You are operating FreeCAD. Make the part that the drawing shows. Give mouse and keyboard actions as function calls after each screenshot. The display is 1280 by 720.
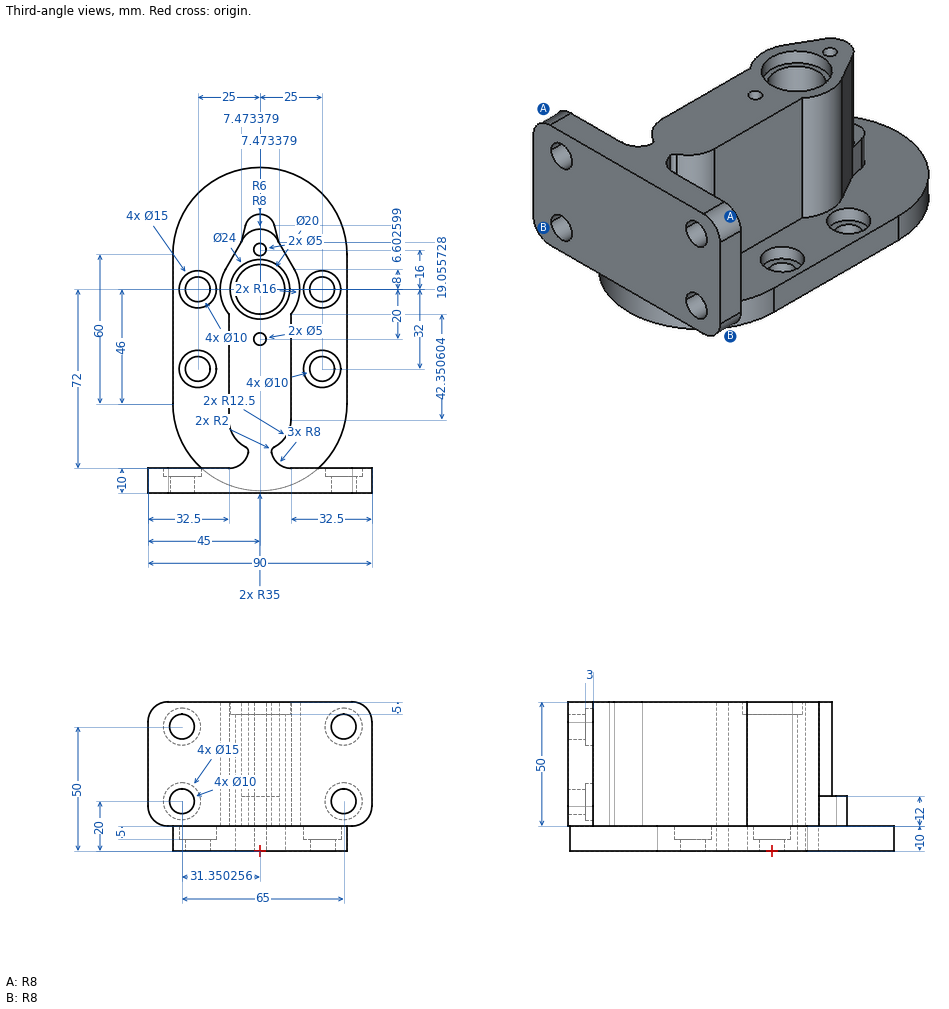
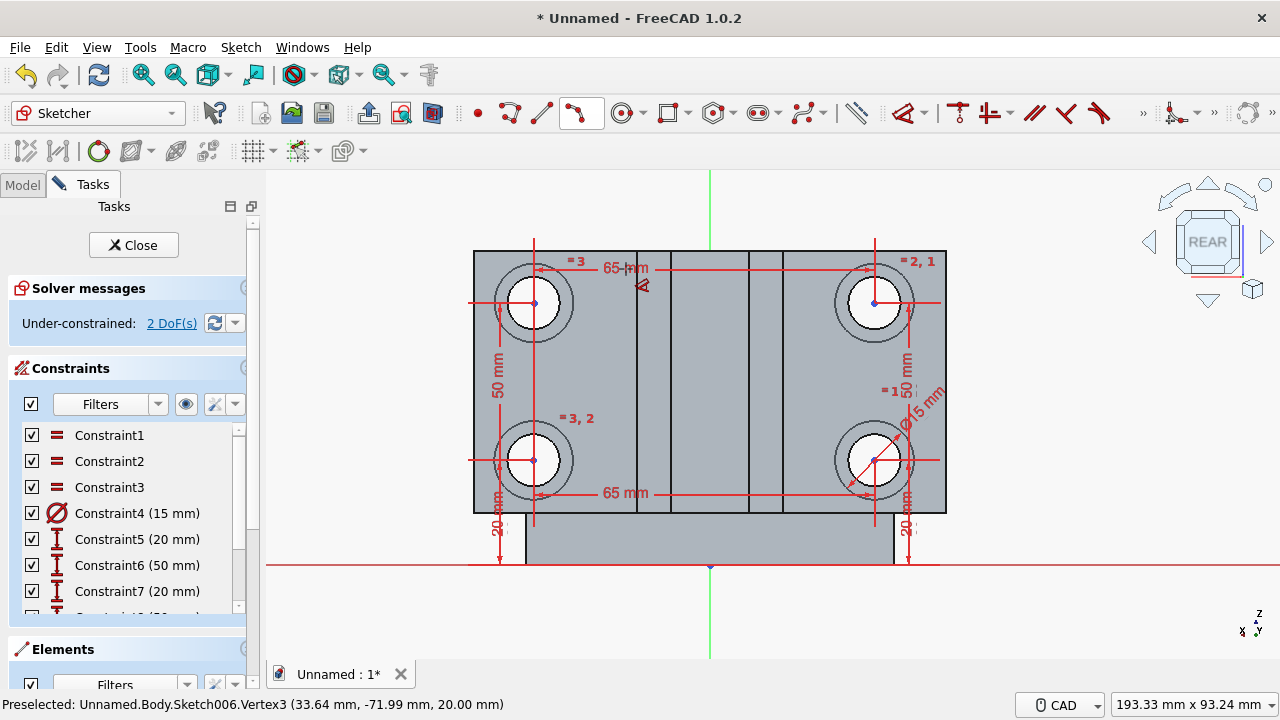
click(875, 303)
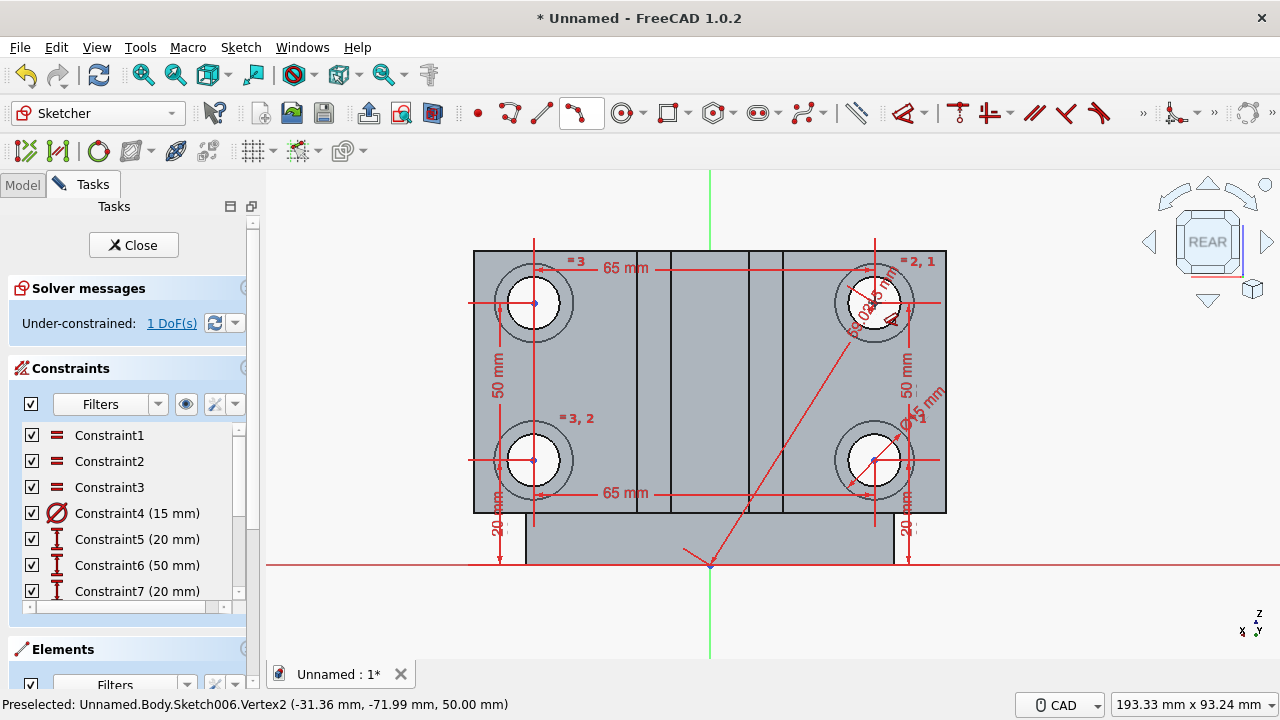
click(534, 303)
click(783, 269)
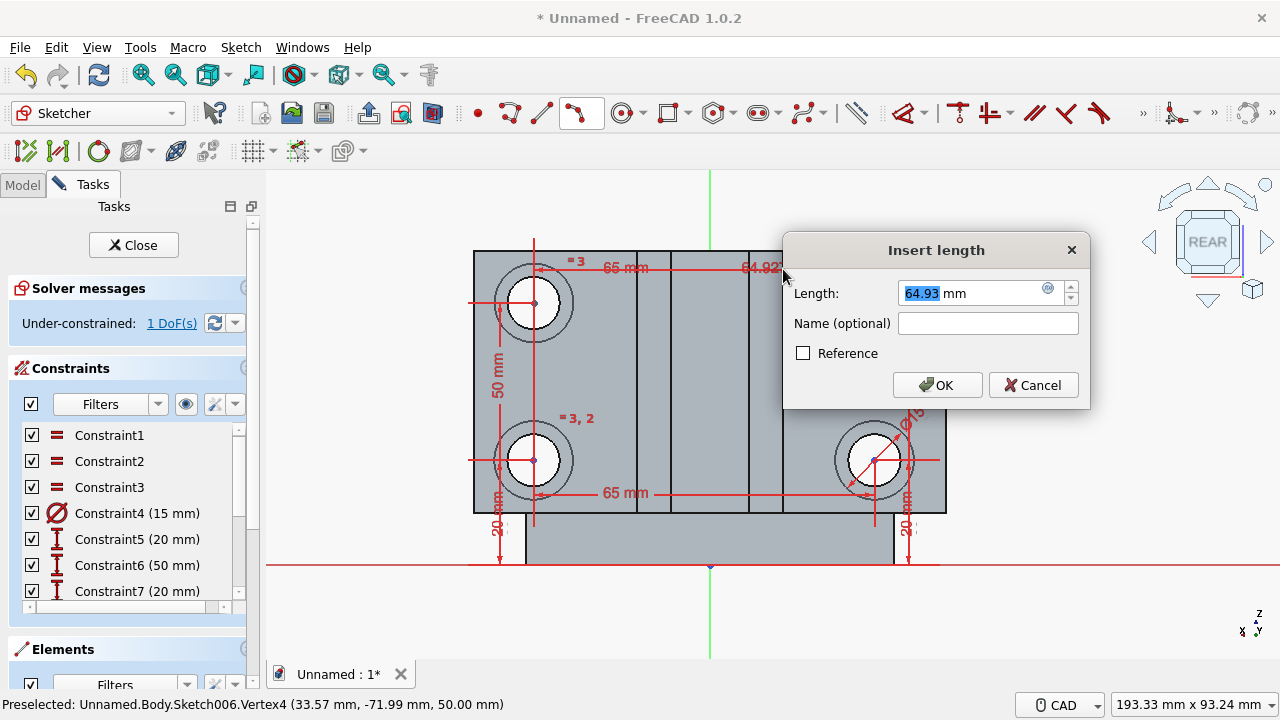
text(65)
key(Return)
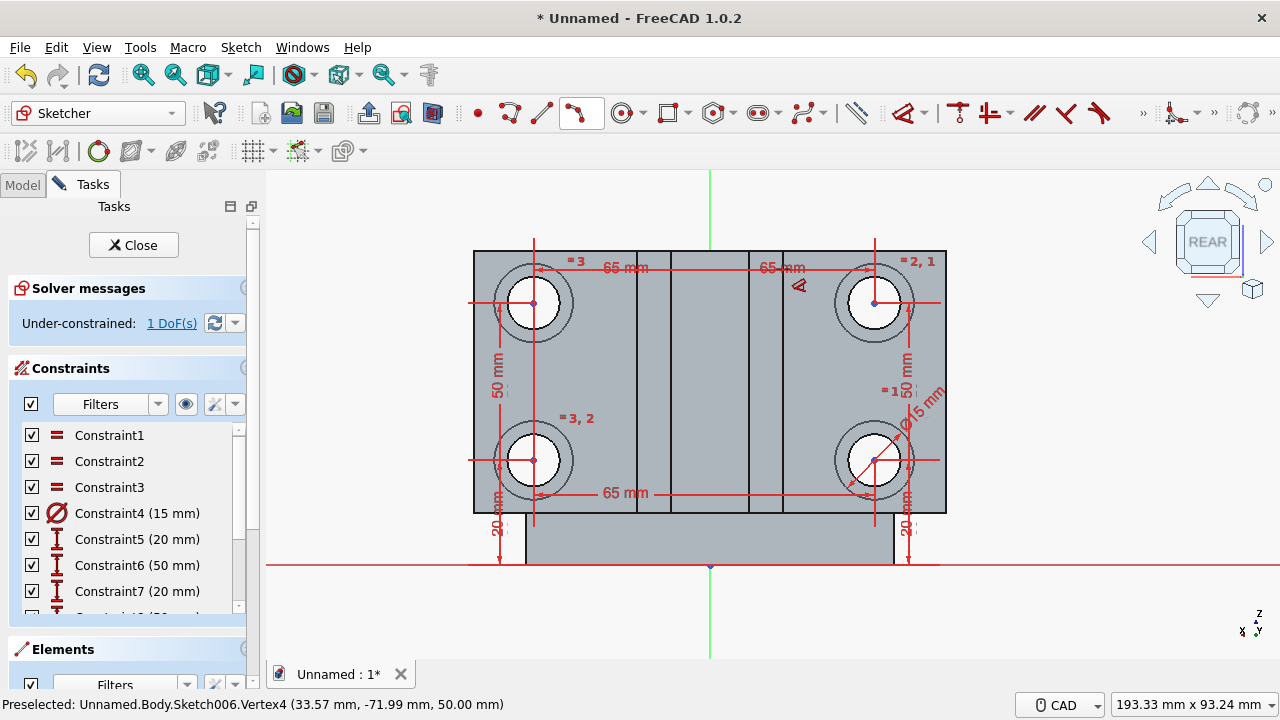
click(875, 460)
click(792, 599)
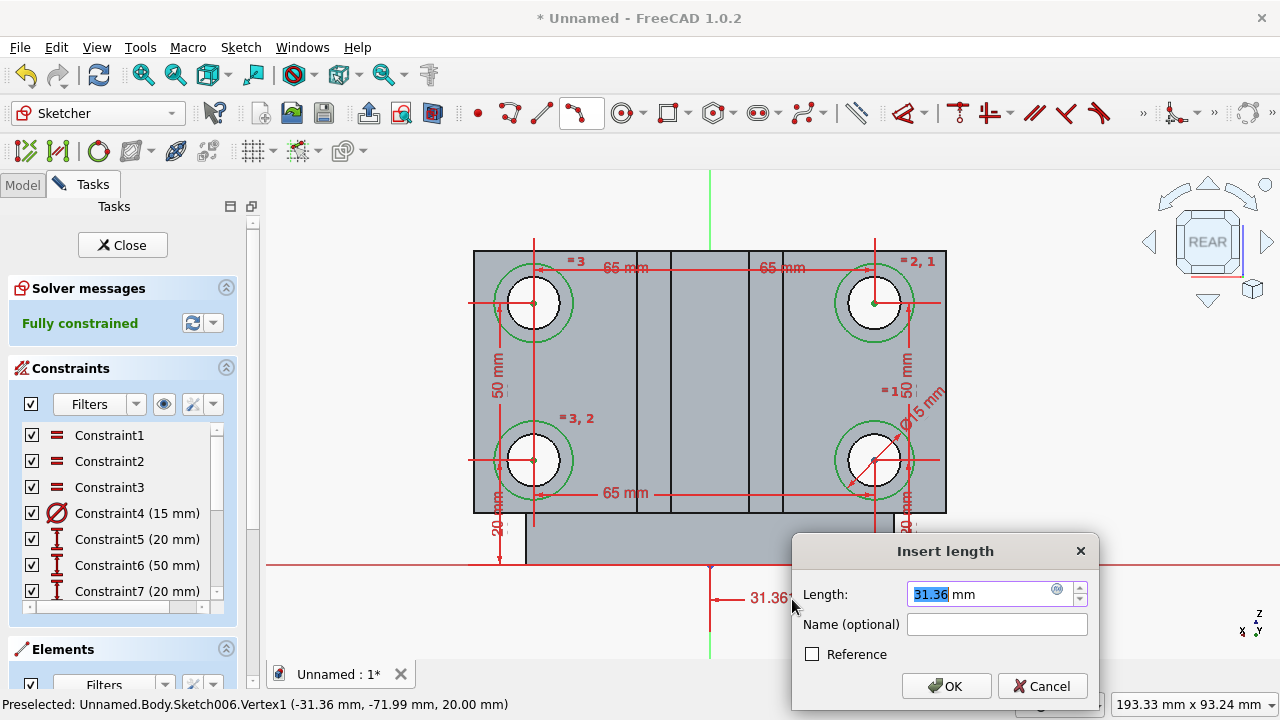
text(31.350256)
key(Return)
key(Escape)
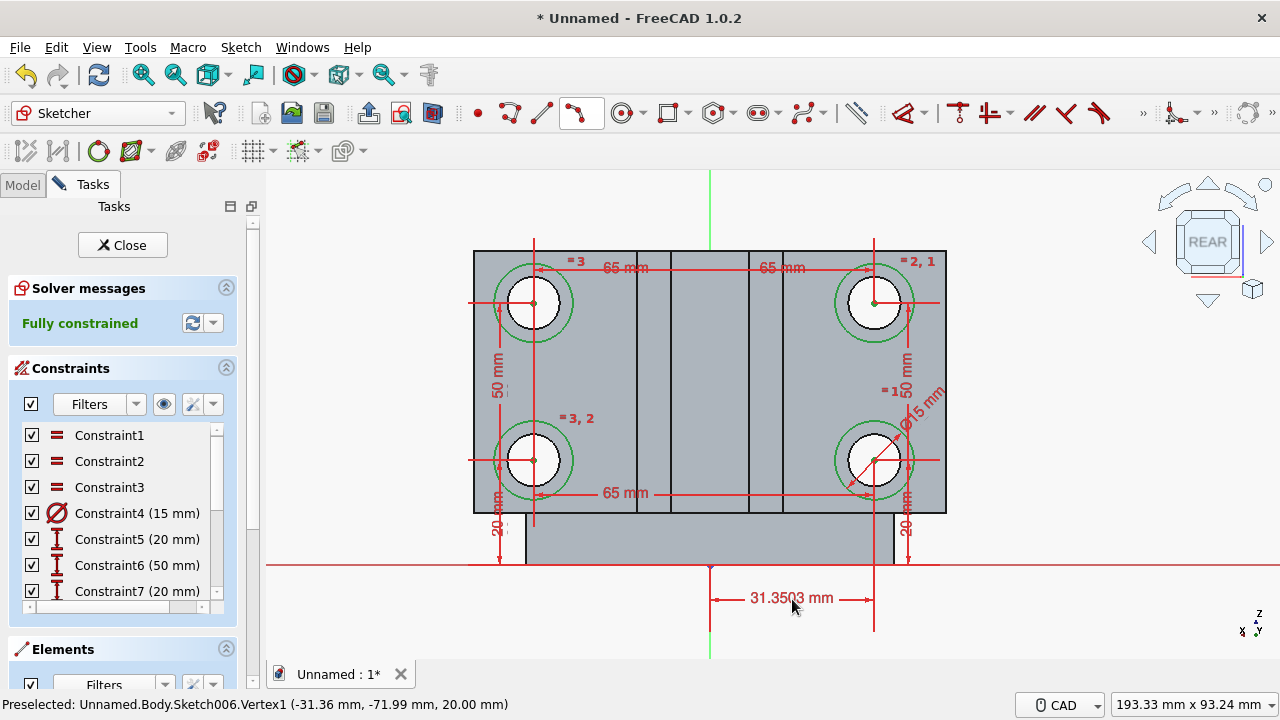
click(123, 245)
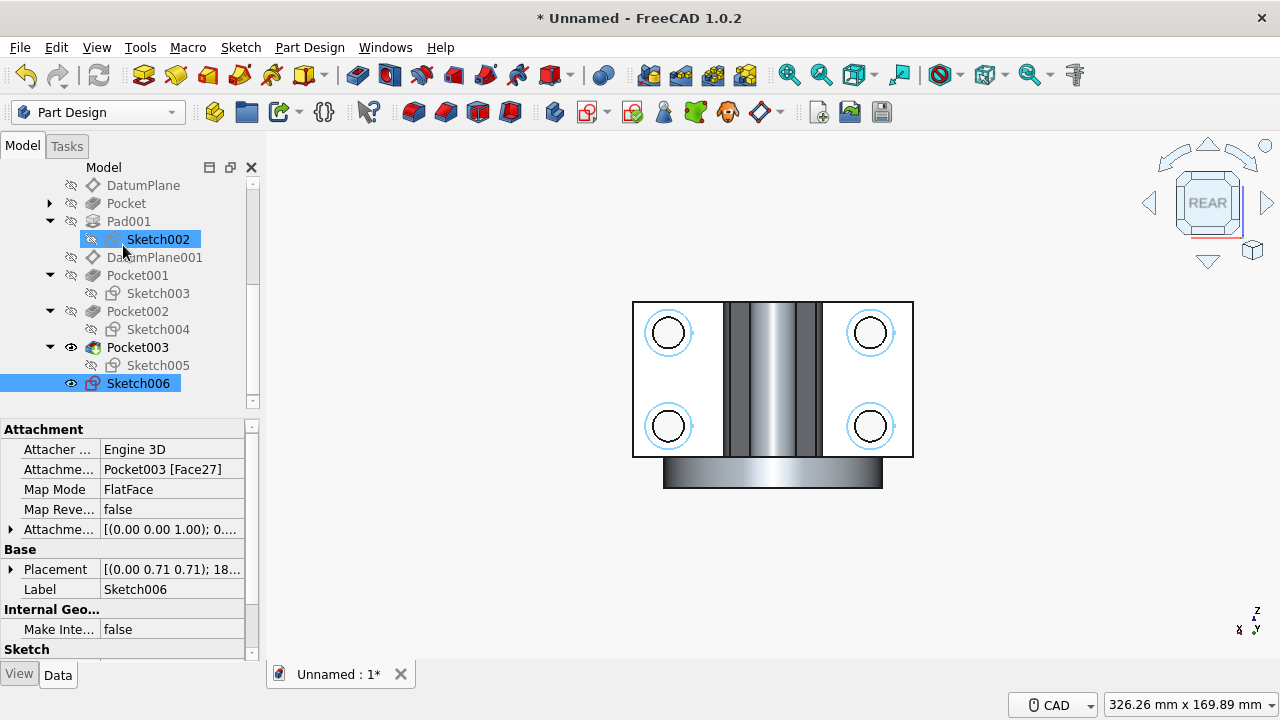
click(358, 76)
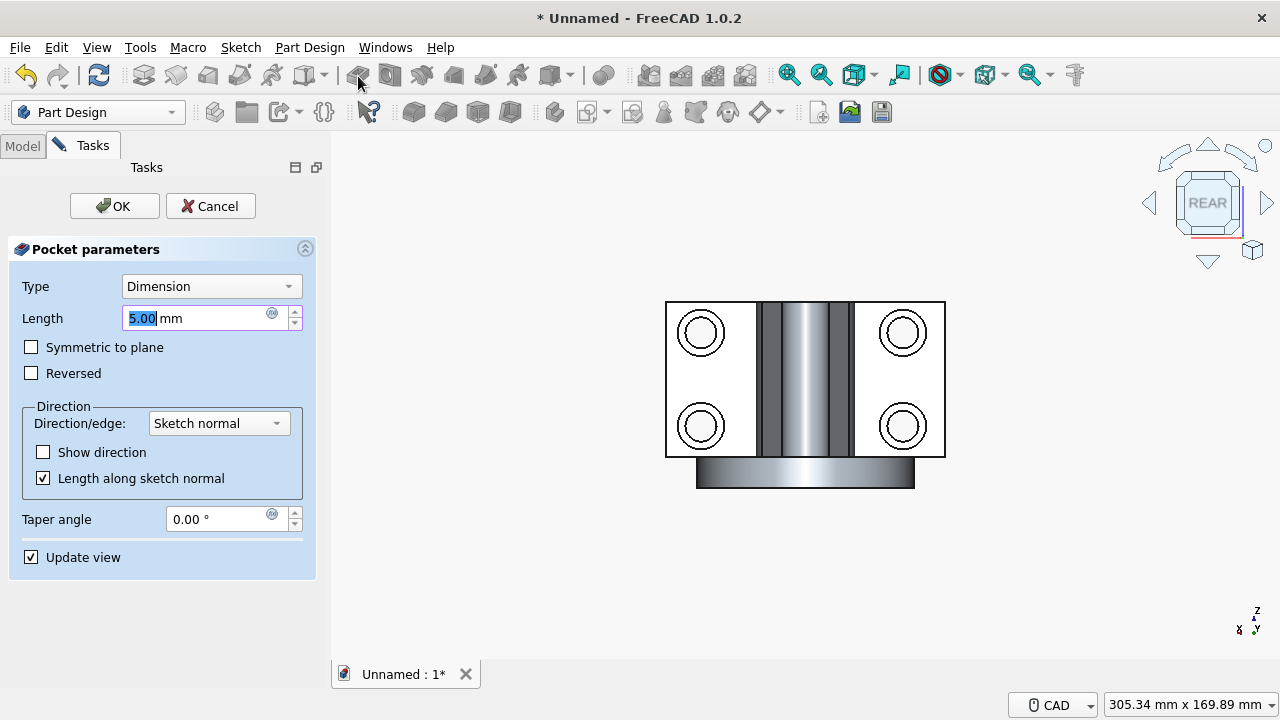
text(3)
key(Tab)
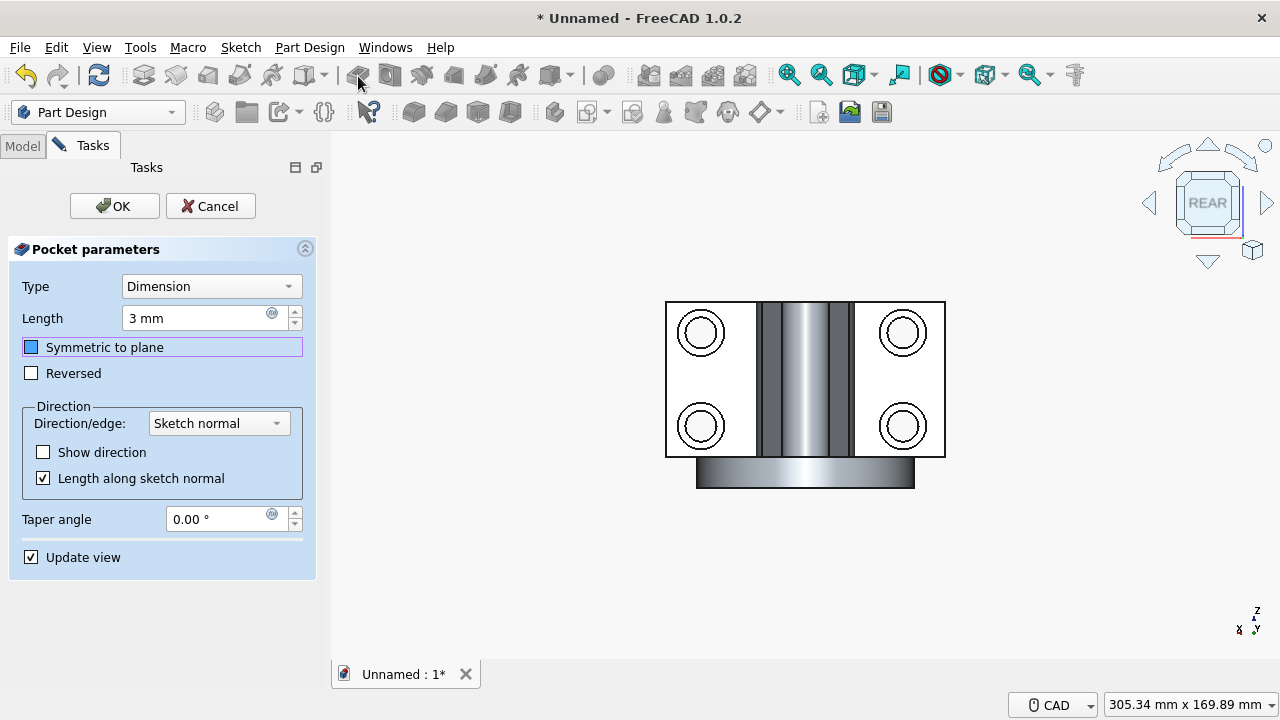
click(115, 206)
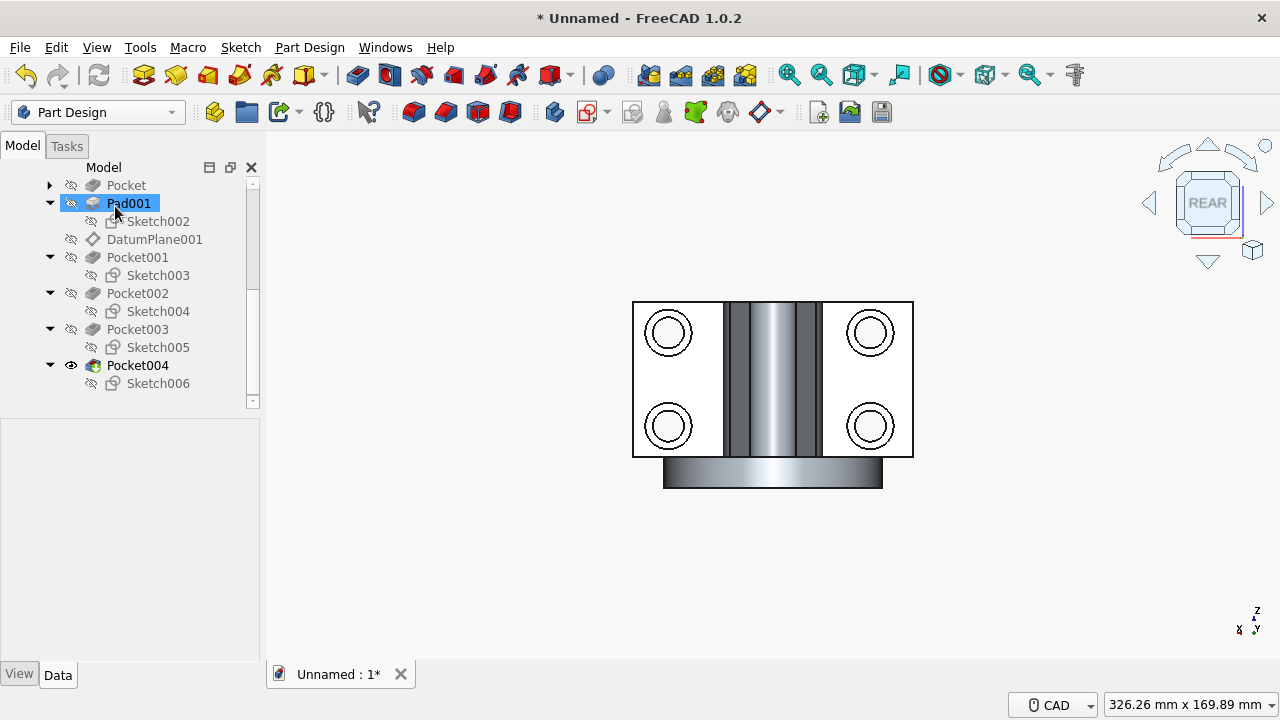
click(790, 76)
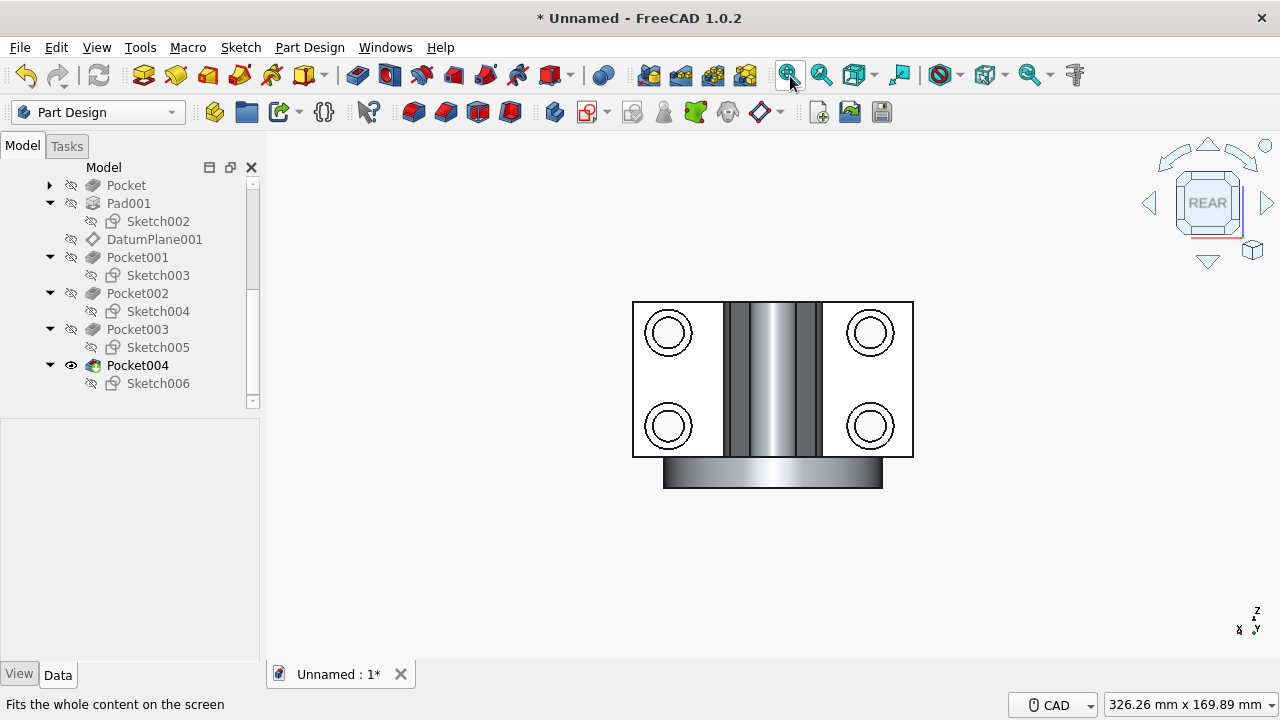
key(0)